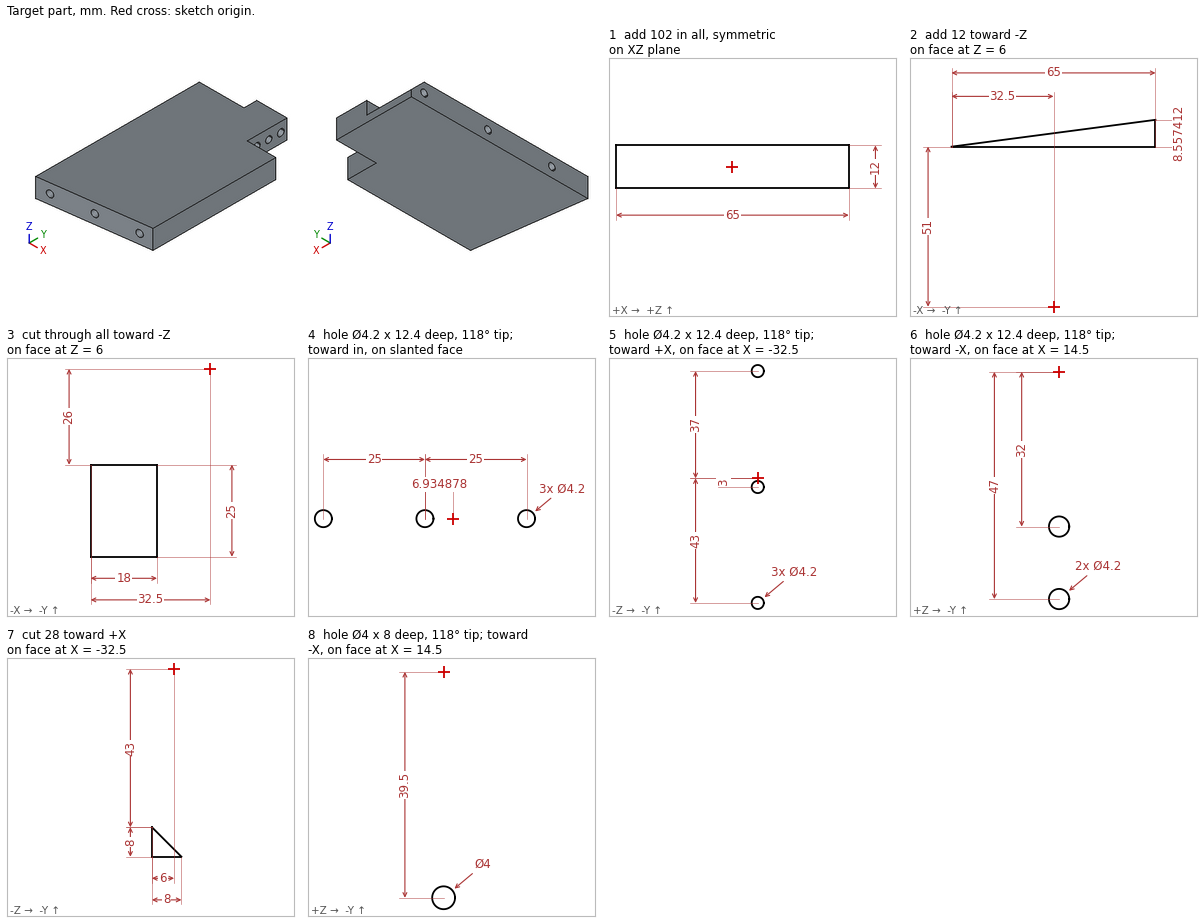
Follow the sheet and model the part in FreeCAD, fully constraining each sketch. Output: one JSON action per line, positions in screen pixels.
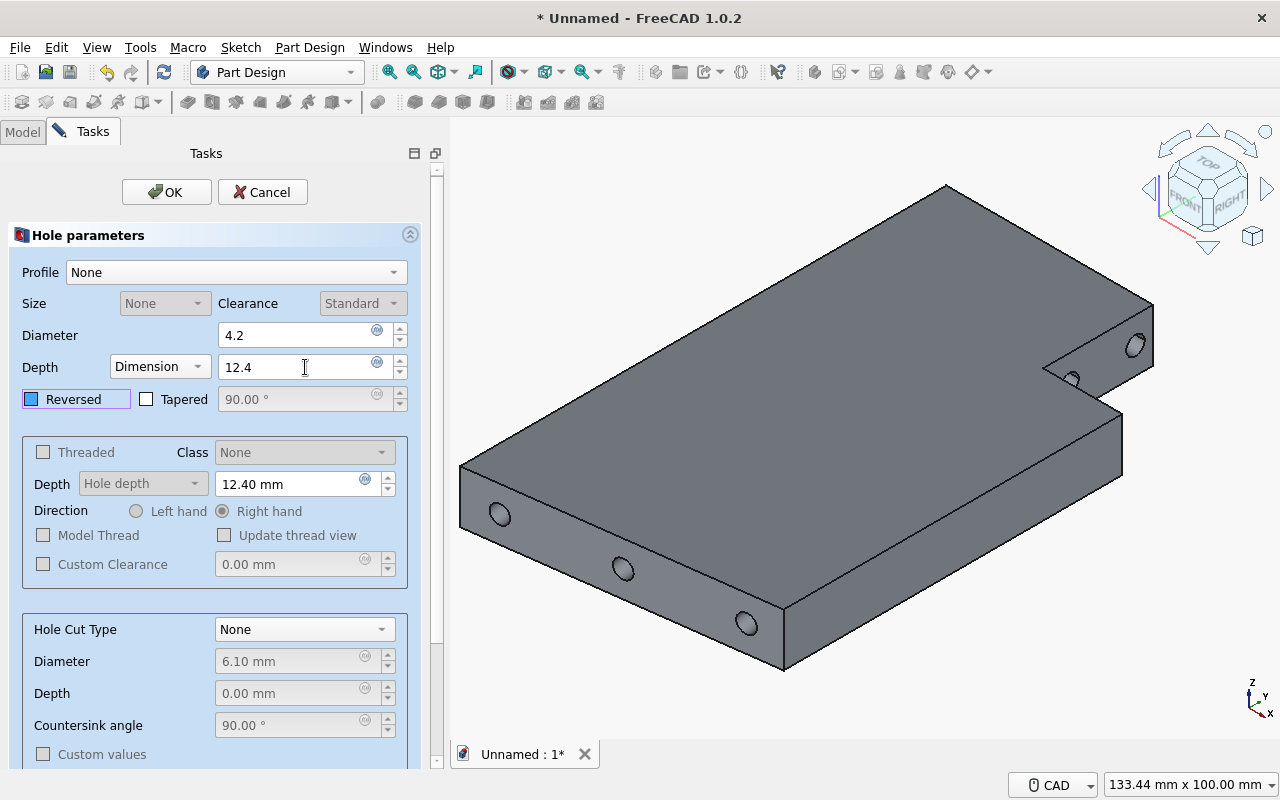
{"action": "left_click", "coordinate": [167, 192]}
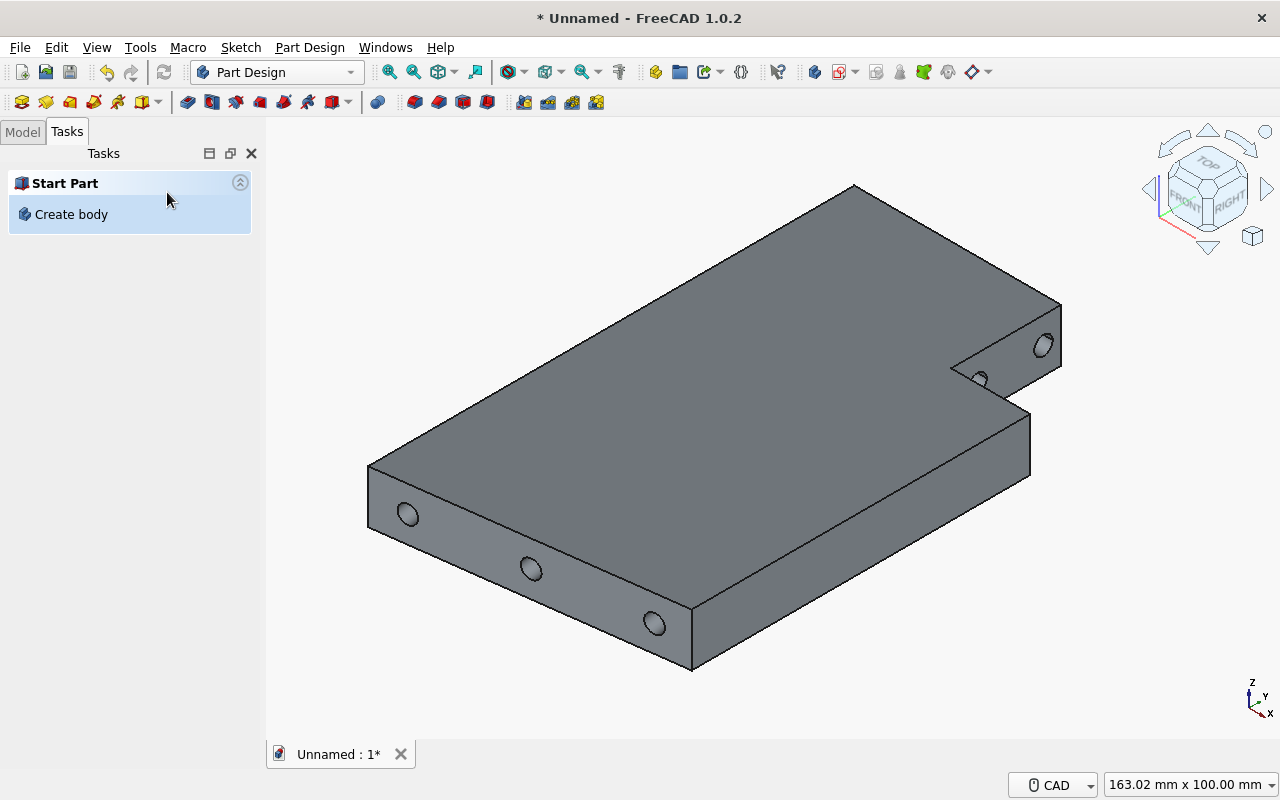
{"action": "key", "text": "6"}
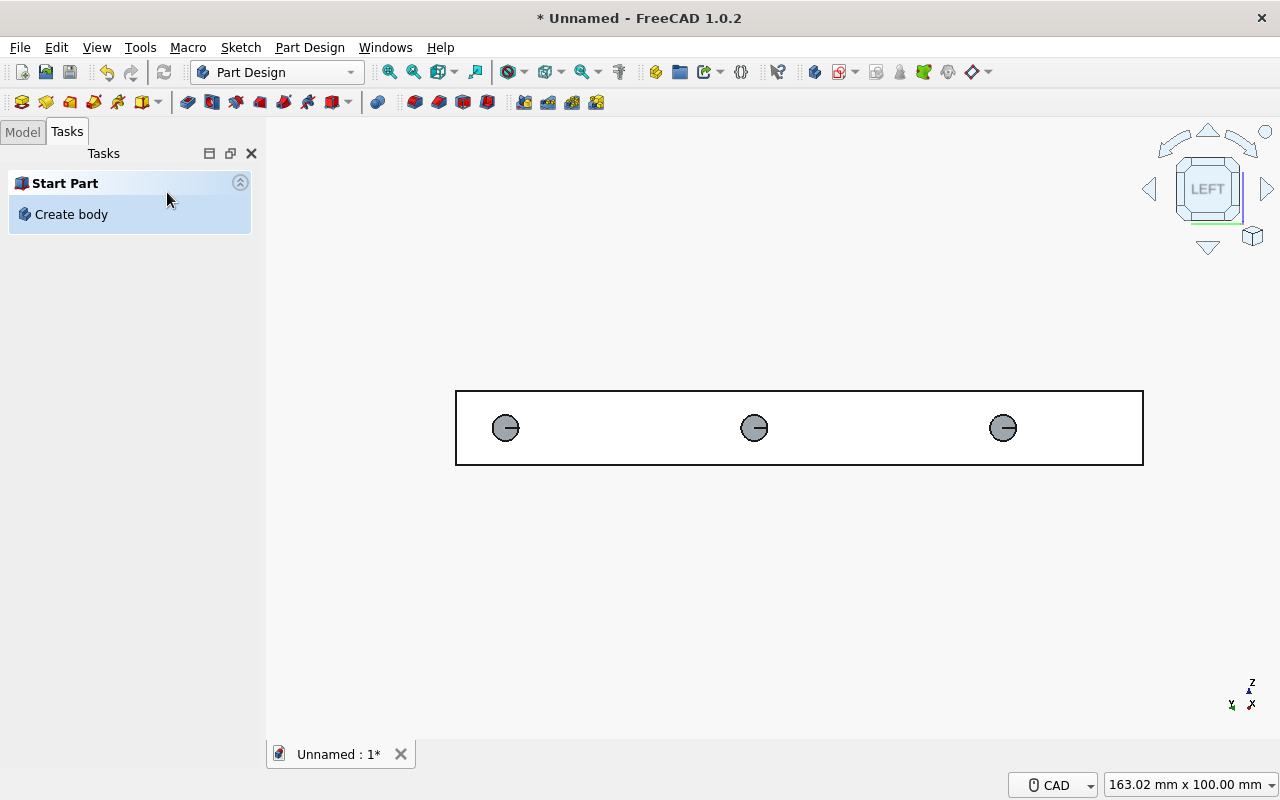
{"action": "left_click", "coordinate": [603, 427]}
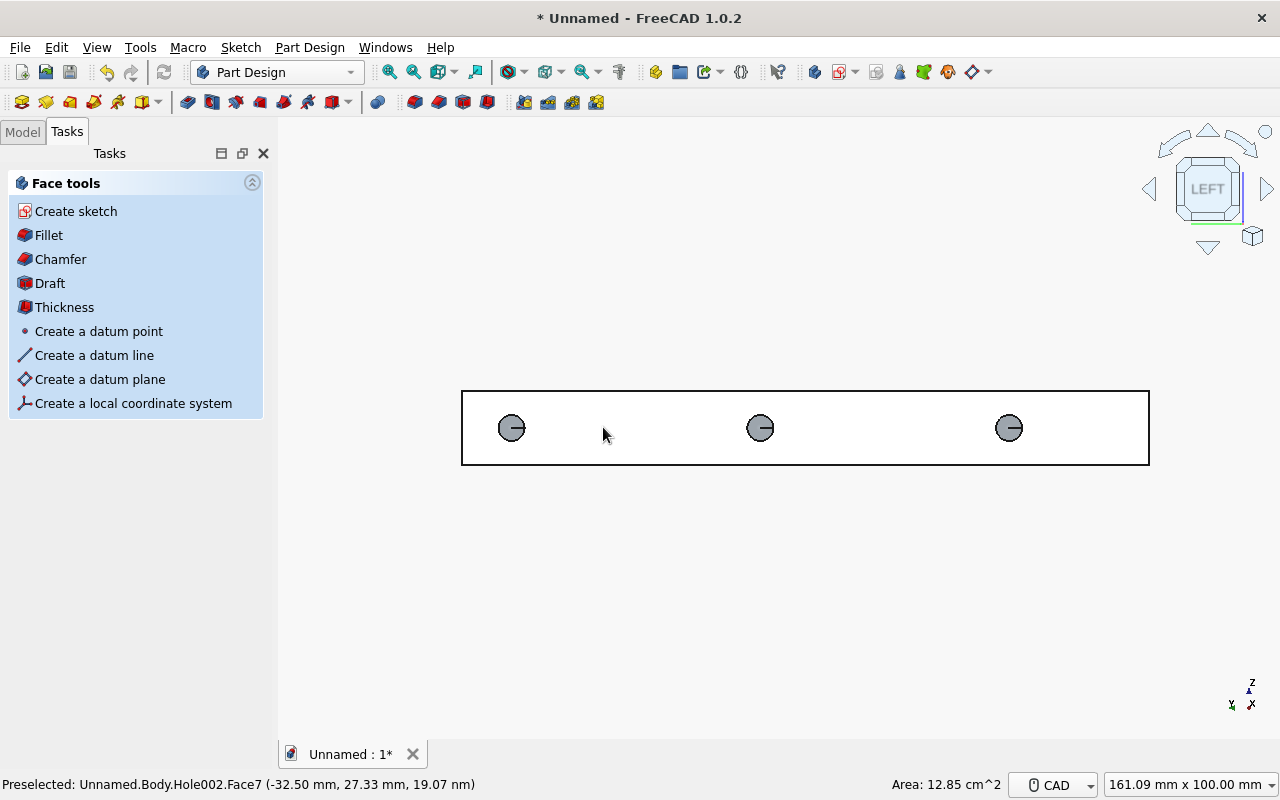
{"action": "left_click", "coordinate": [840, 72]}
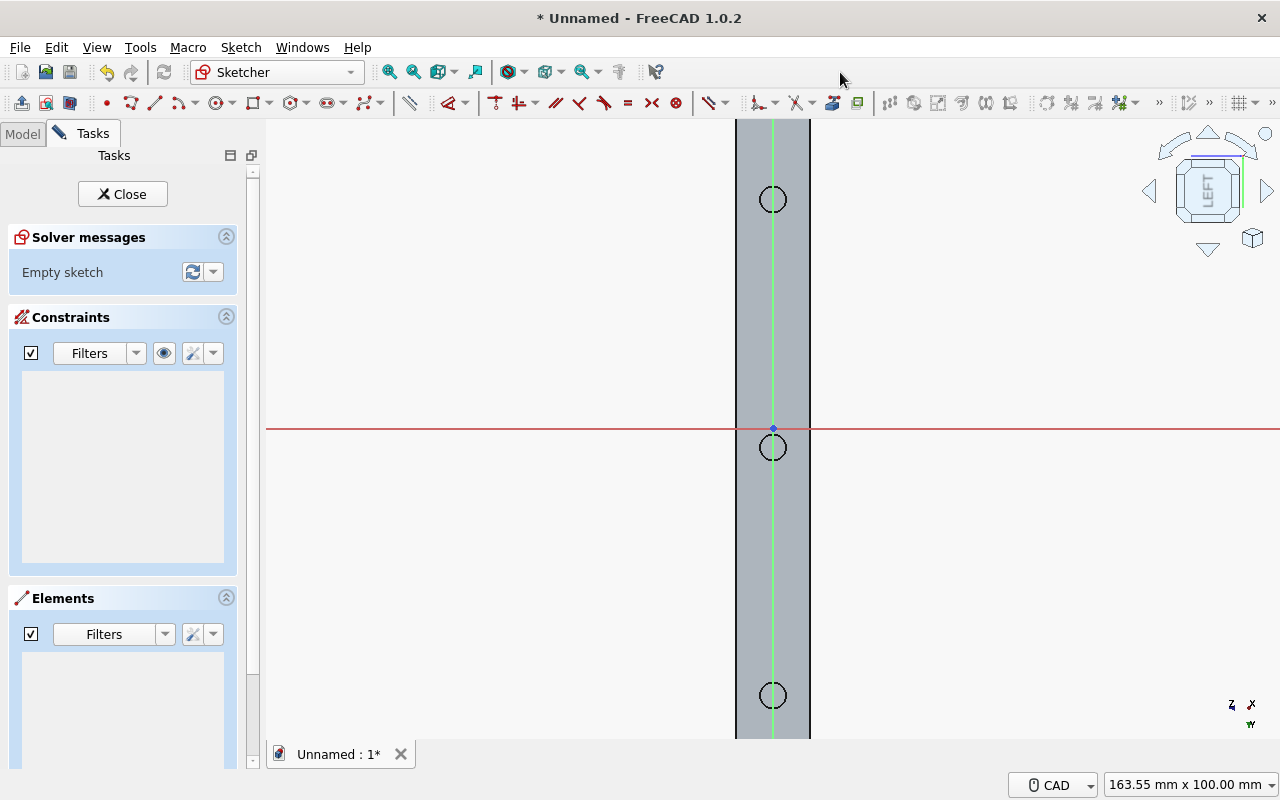
{"action": "scroll", "coordinate": [704, 429], "scroll_direction": "down", "scroll_amount": 5}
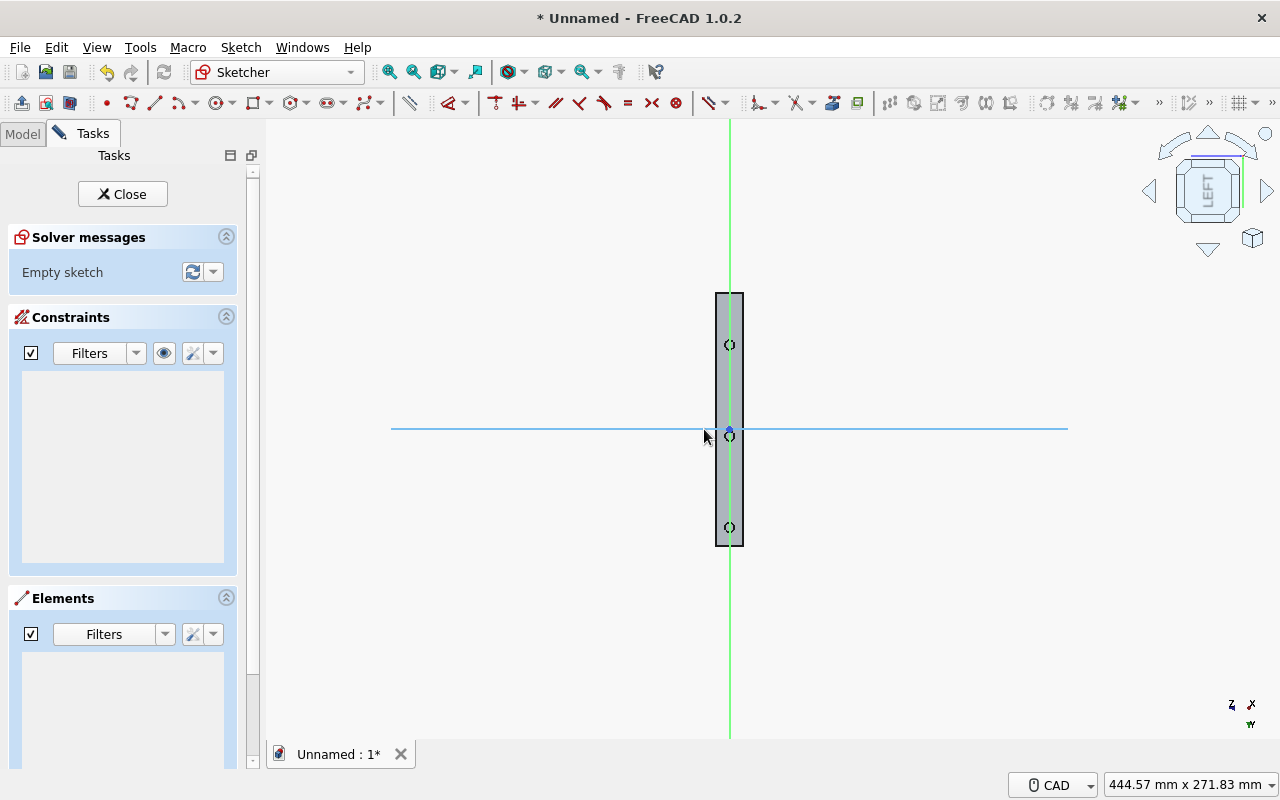
{"action": "scroll", "coordinate": [726, 542], "scroll_direction": "up", "scroll_amount": 15}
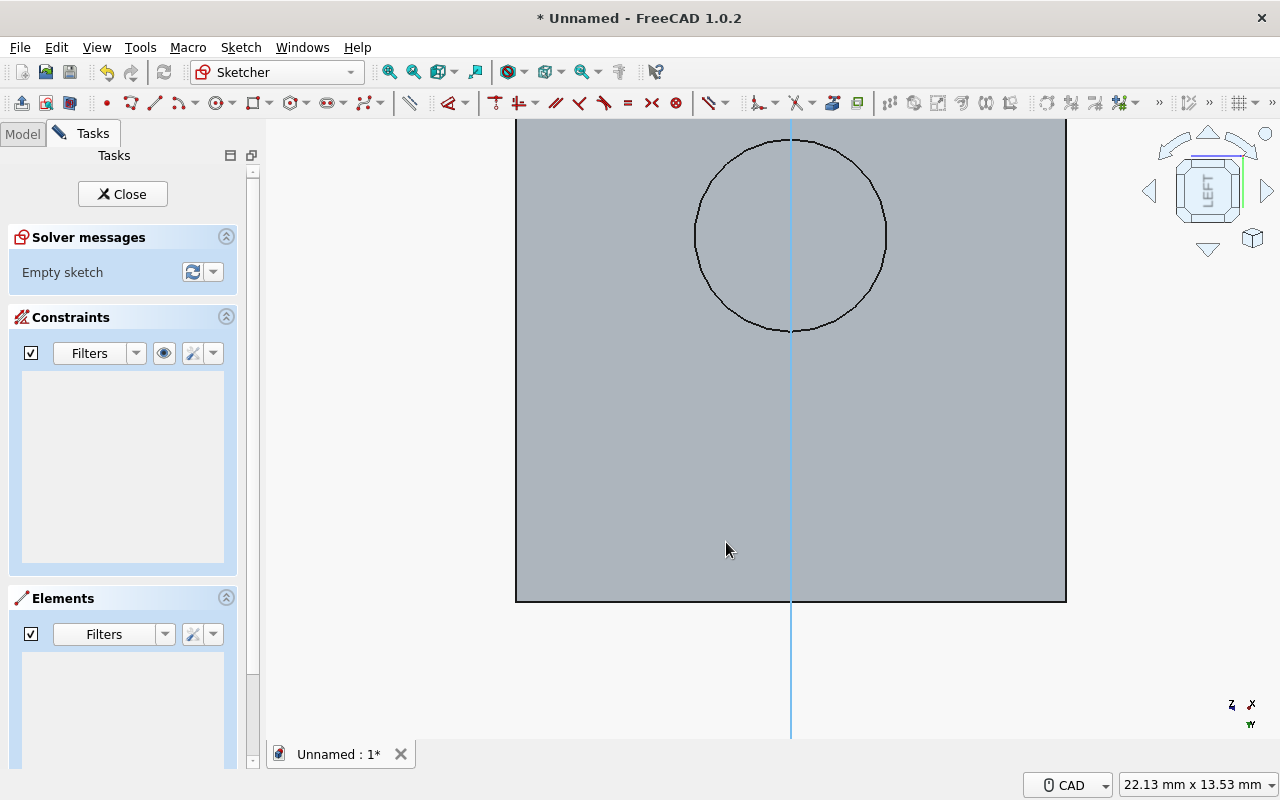
{"action": "left_click", "coordinate": [132, 104]}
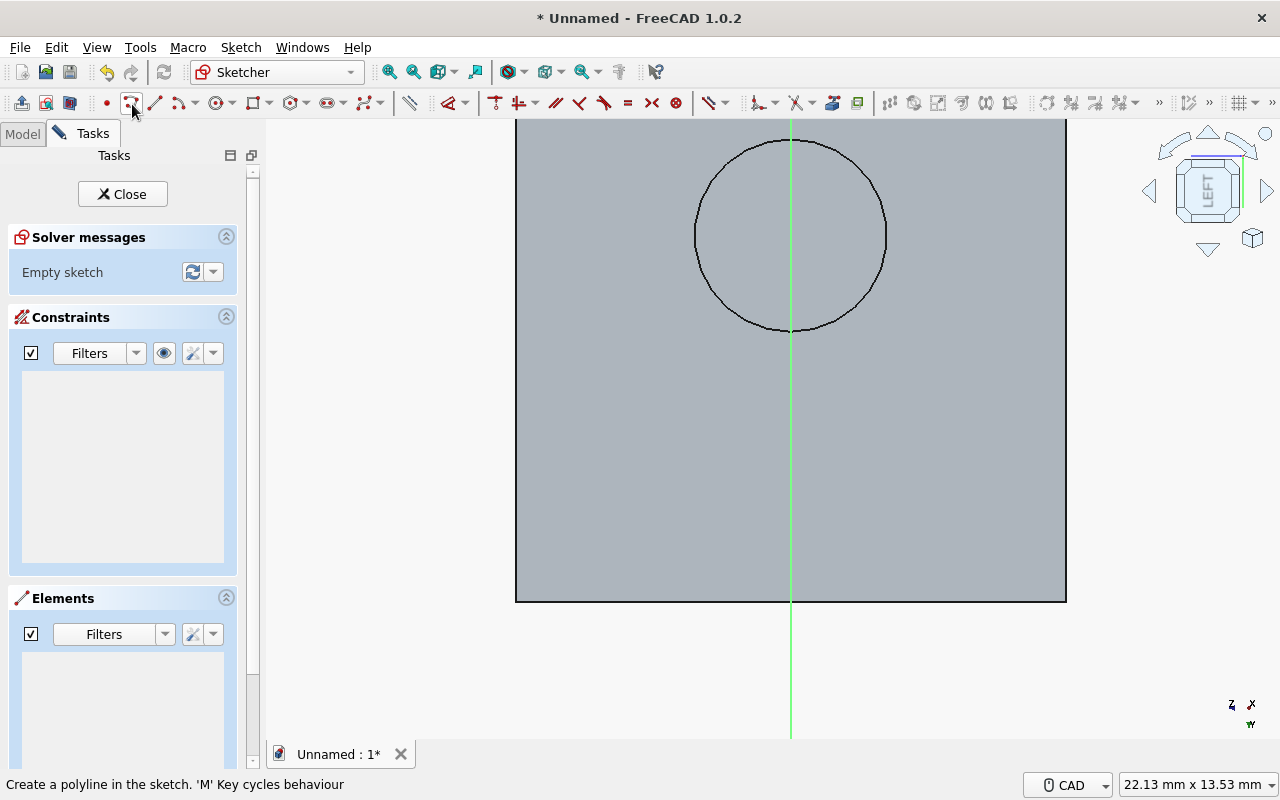
{"action": "left_click", "coordinate": [516, 236]}
{"action": "left_click", "coordinate": [516, 602]}
{"action": "left_click", "coordinate": [882, 602]}
{"action": "left_click", "coordinate": [516, 237]}
{"action": "key", "text": "Escape"}
{"action": "key", "text": "Escape"}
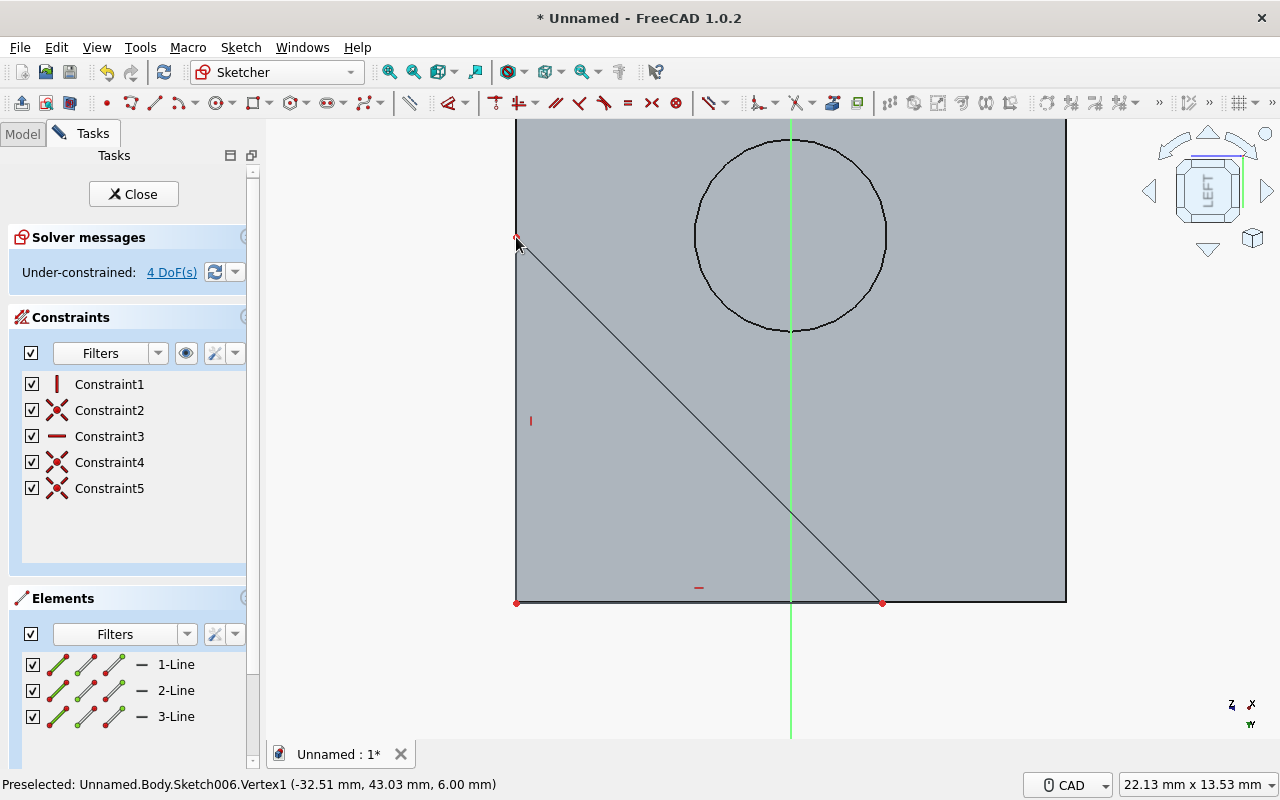
{"action": "key", "text": "d"}